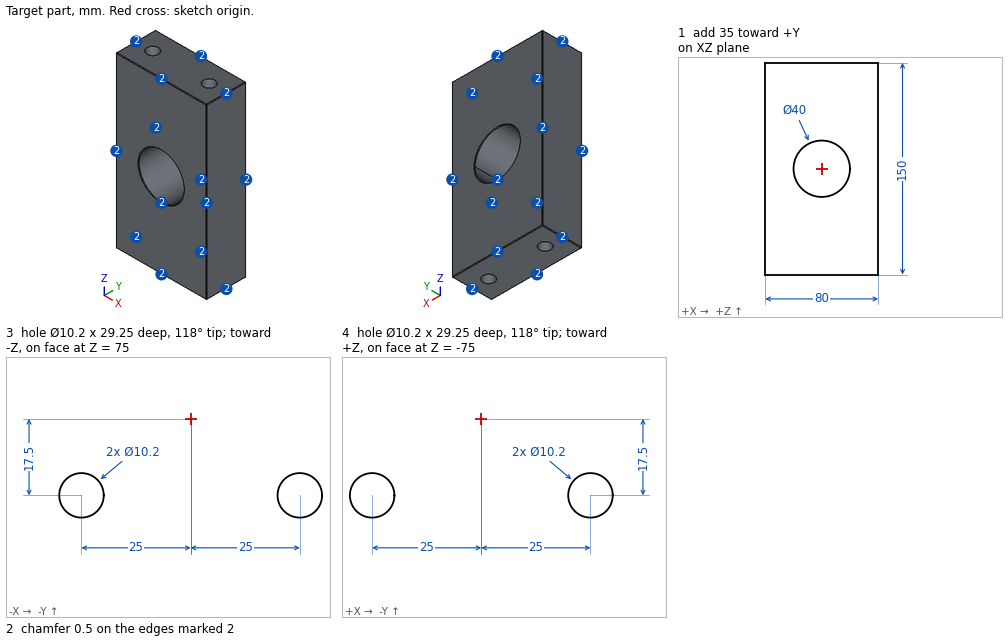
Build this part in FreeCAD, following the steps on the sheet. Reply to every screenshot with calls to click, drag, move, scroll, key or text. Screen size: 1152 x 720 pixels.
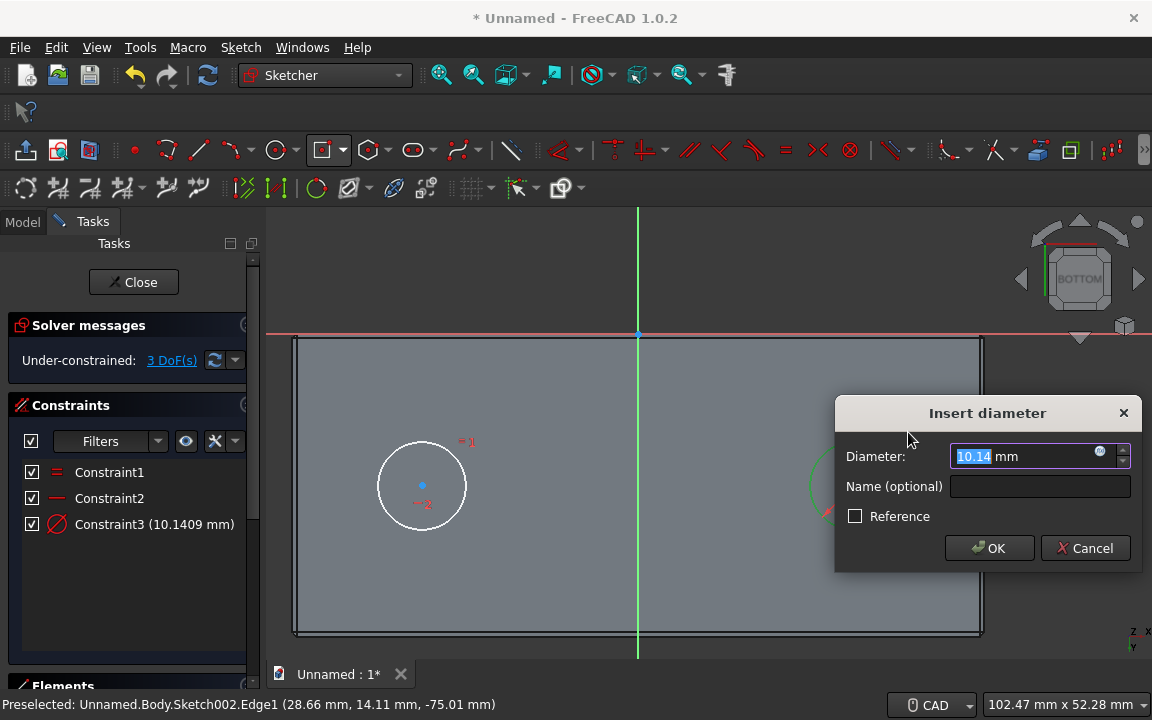
text(10.2)
key(Return)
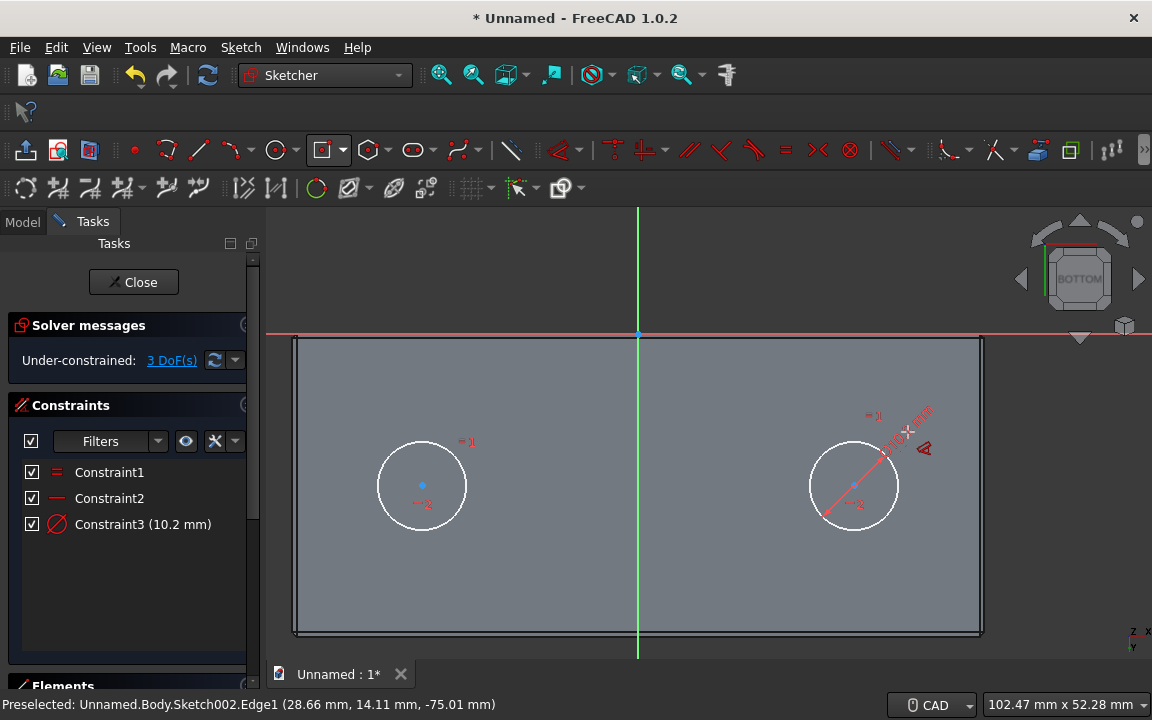
click(854, 486)
click(746, 300)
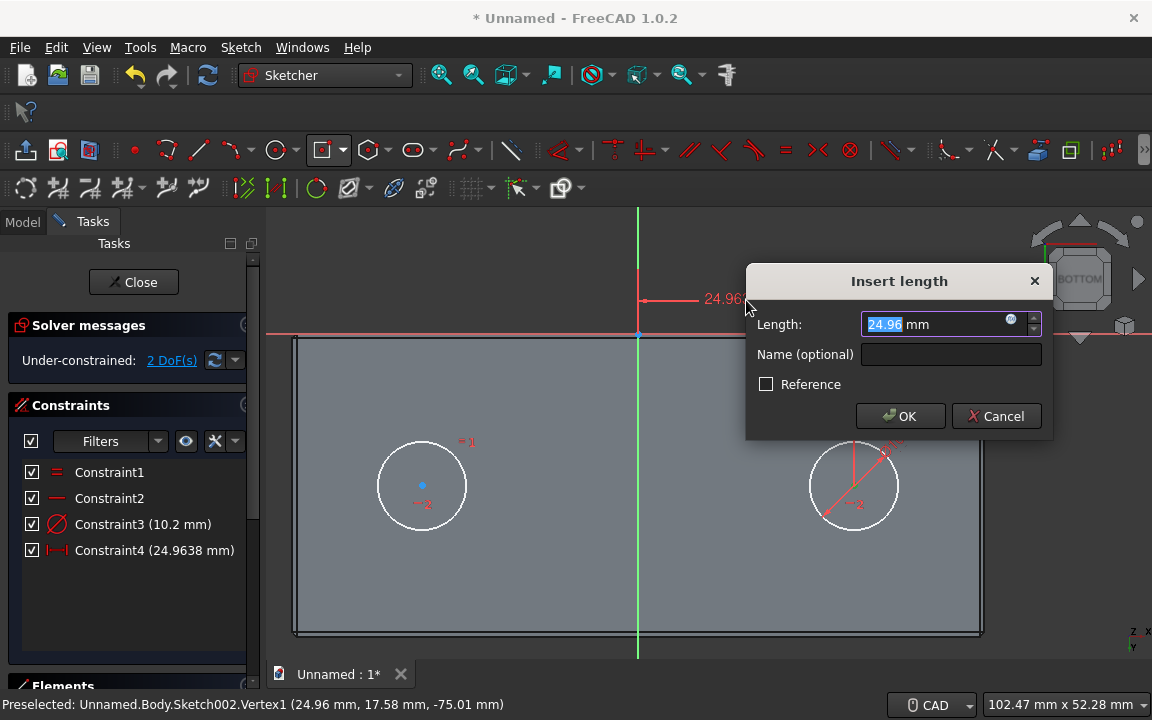
text(25)
key(Return)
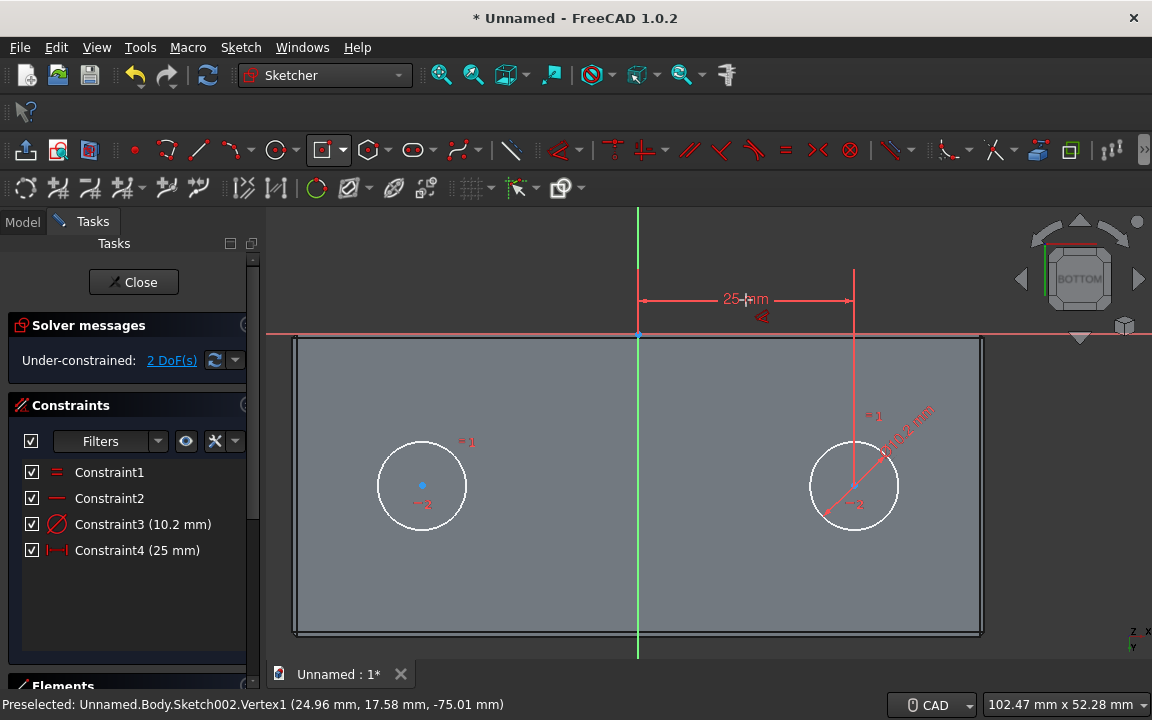
click(422, 486)
click(530, 300)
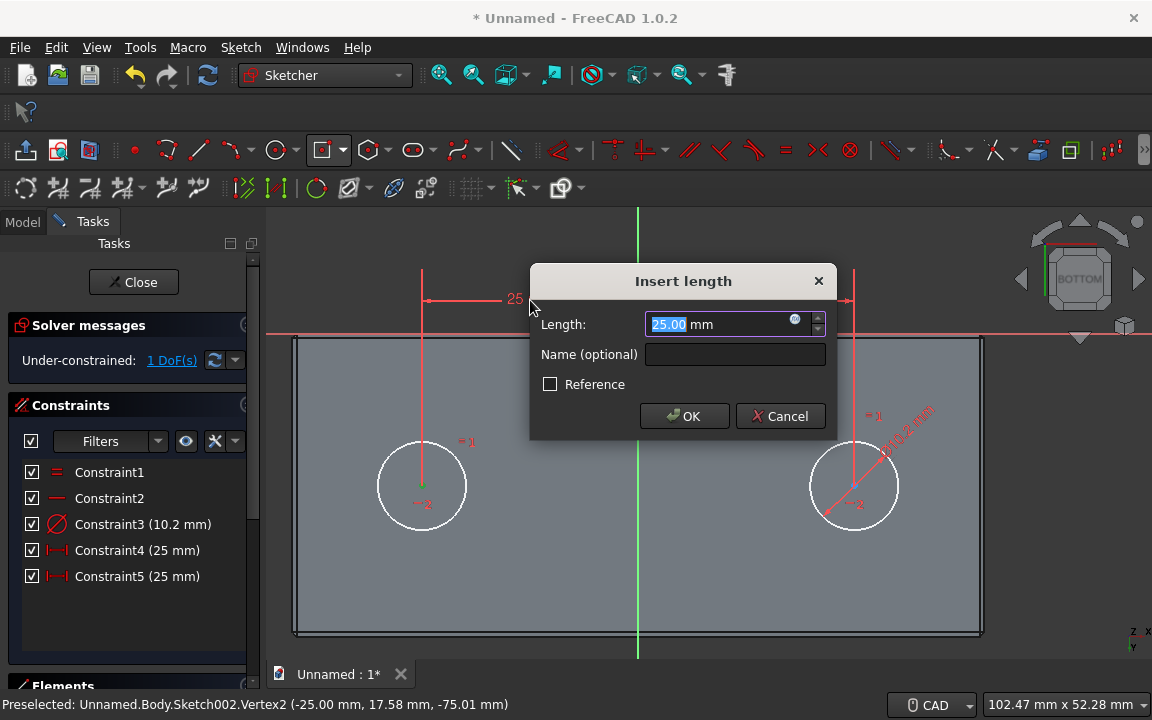
text(25)
key(Return)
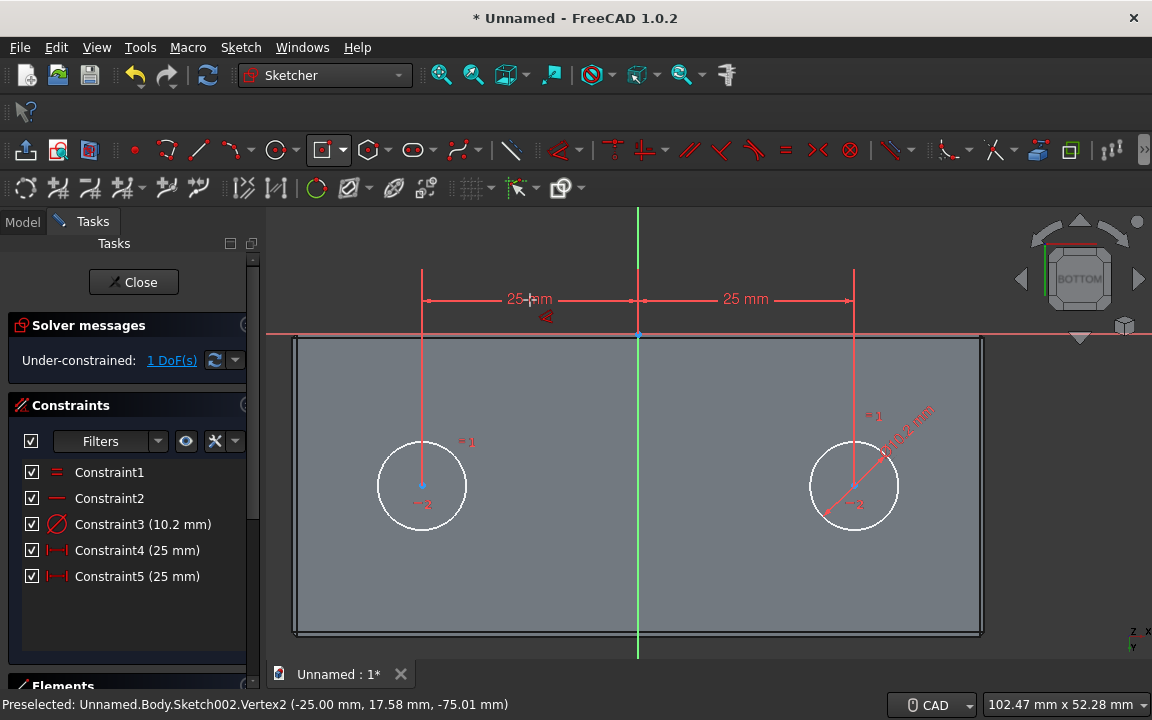
click(854, 486)
click(888, 410)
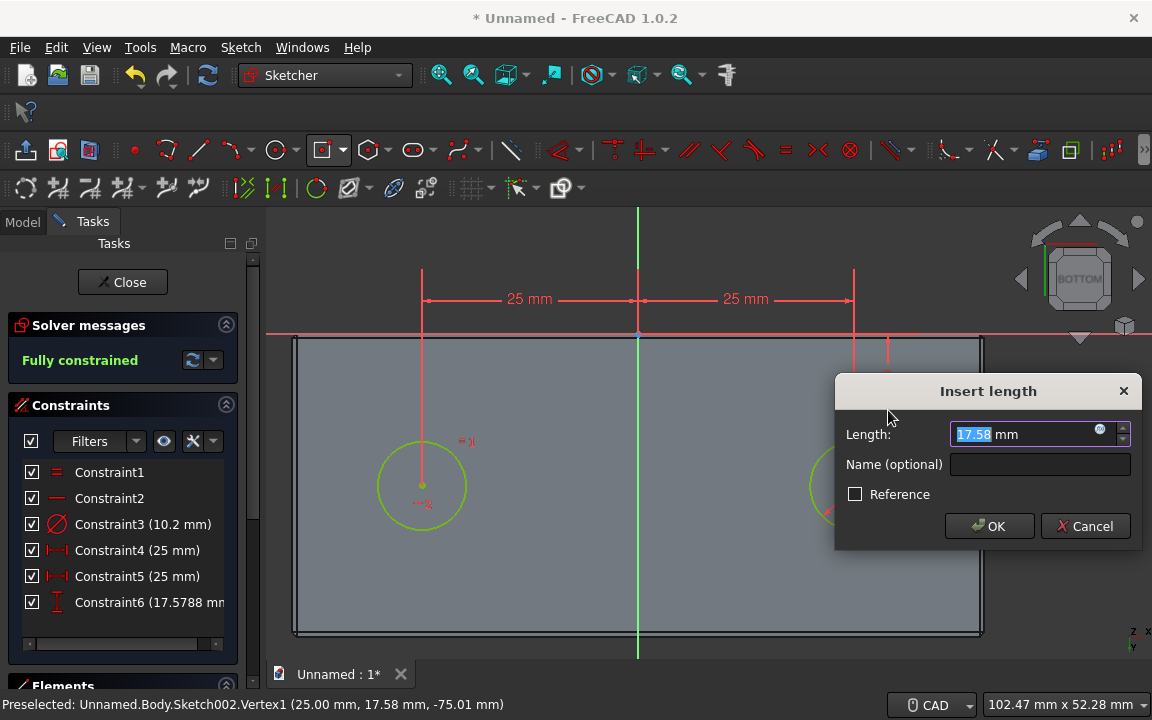
text(17.5)
key(Return)
key(Escape)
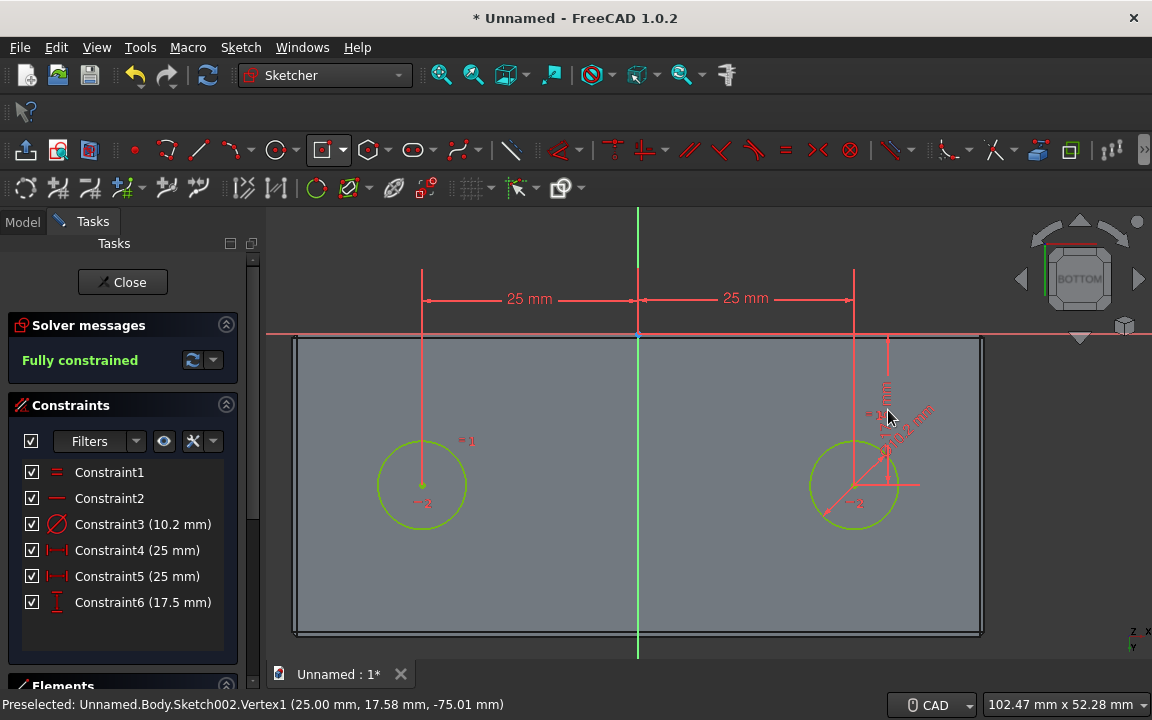
click(123, 282)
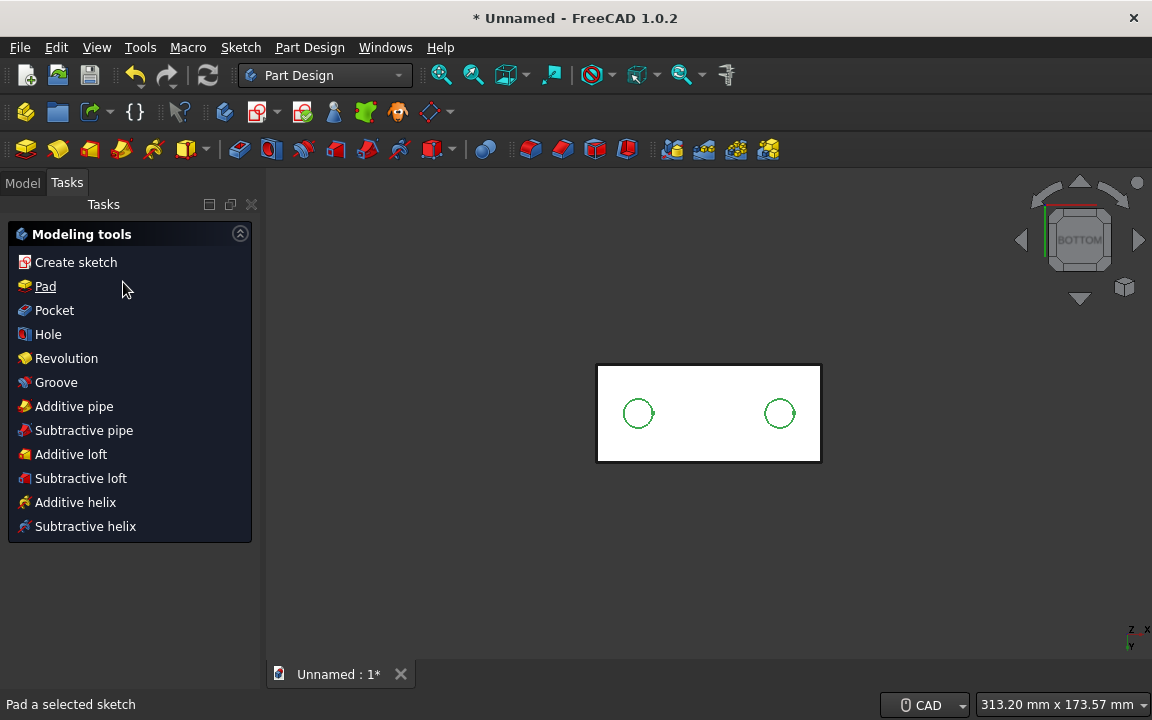
click(272, 150)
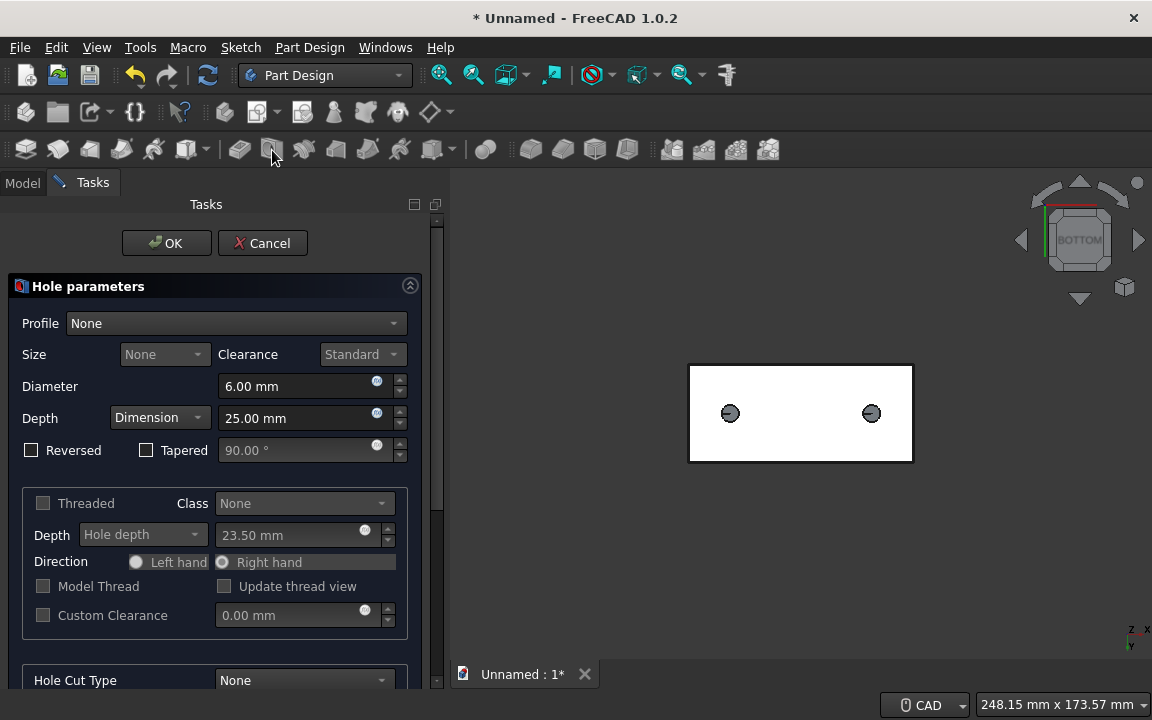
triple_click(305, 386)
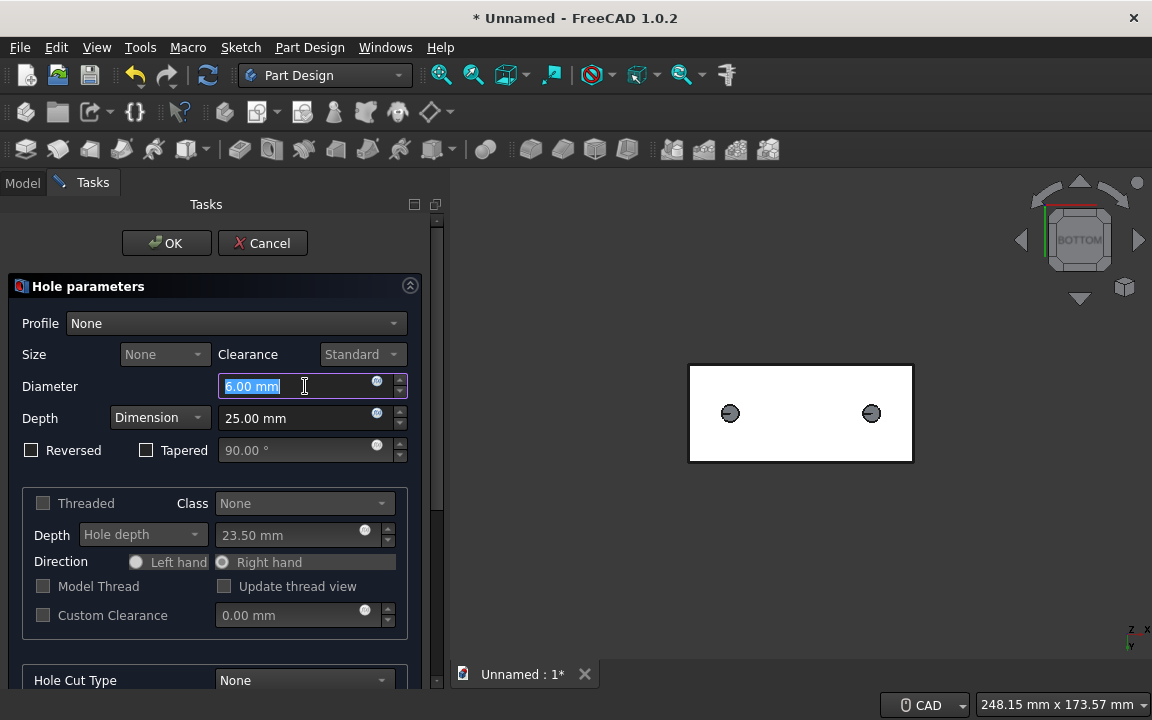
text(10.2)
key(Tab)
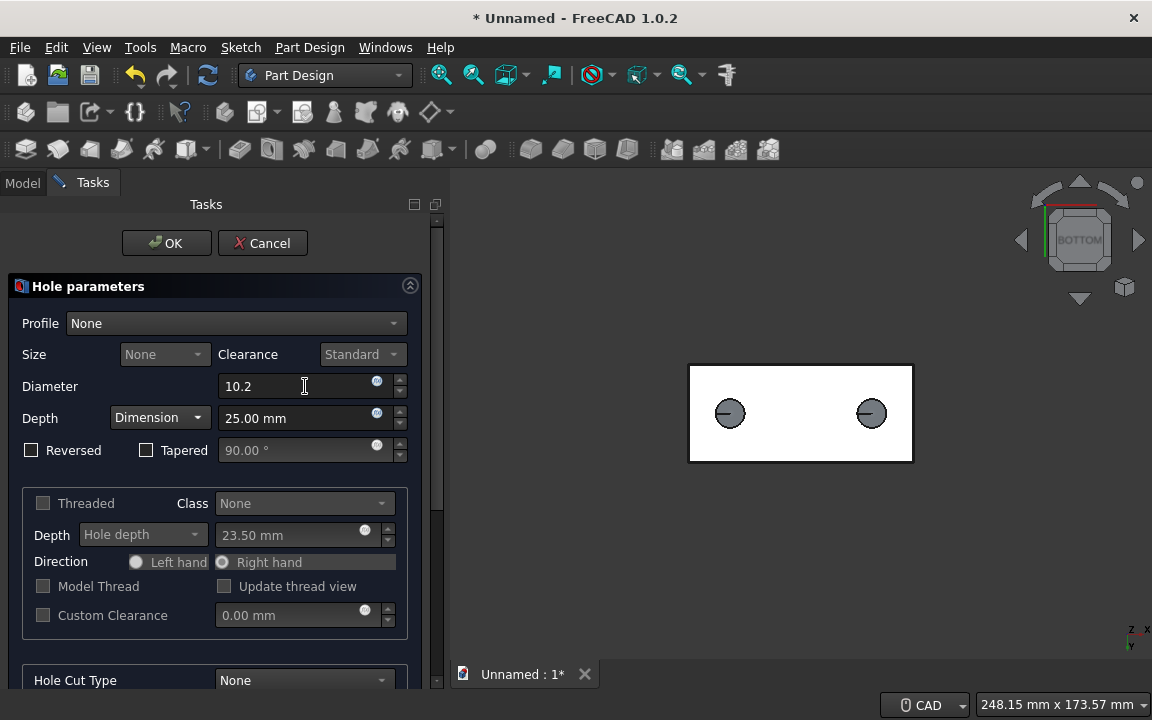
triple_click(305, 418)